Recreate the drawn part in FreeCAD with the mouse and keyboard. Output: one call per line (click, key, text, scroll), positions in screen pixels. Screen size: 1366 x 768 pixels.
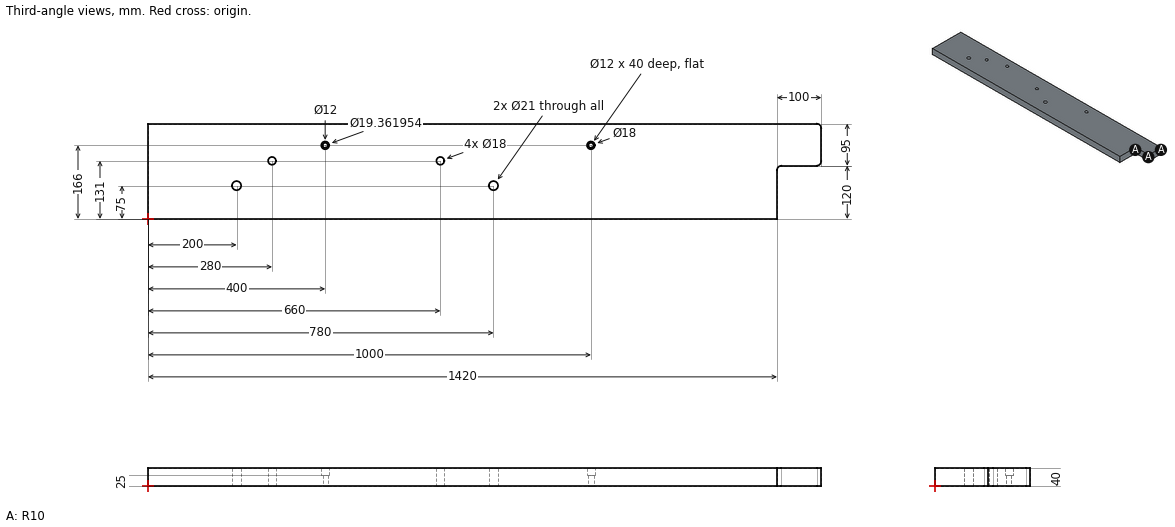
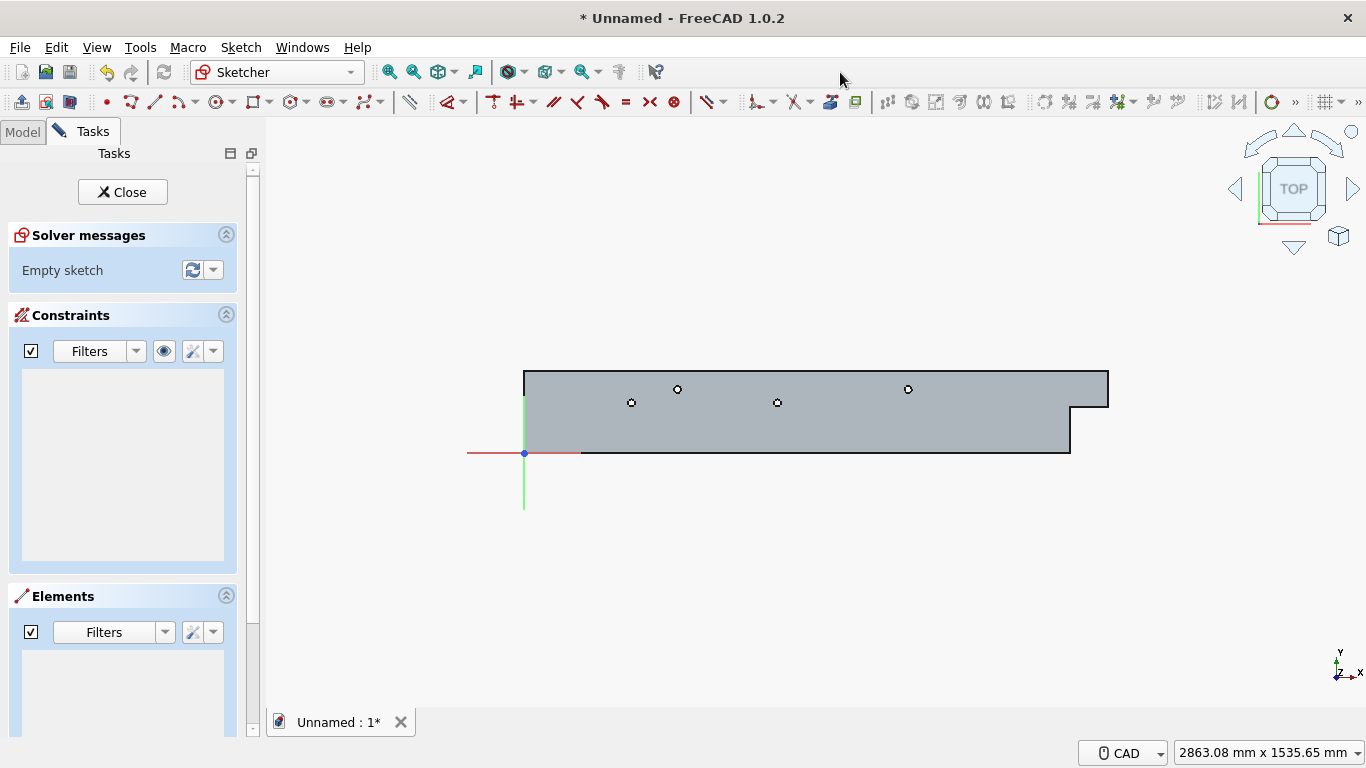
scroll(617, 457, up, 4)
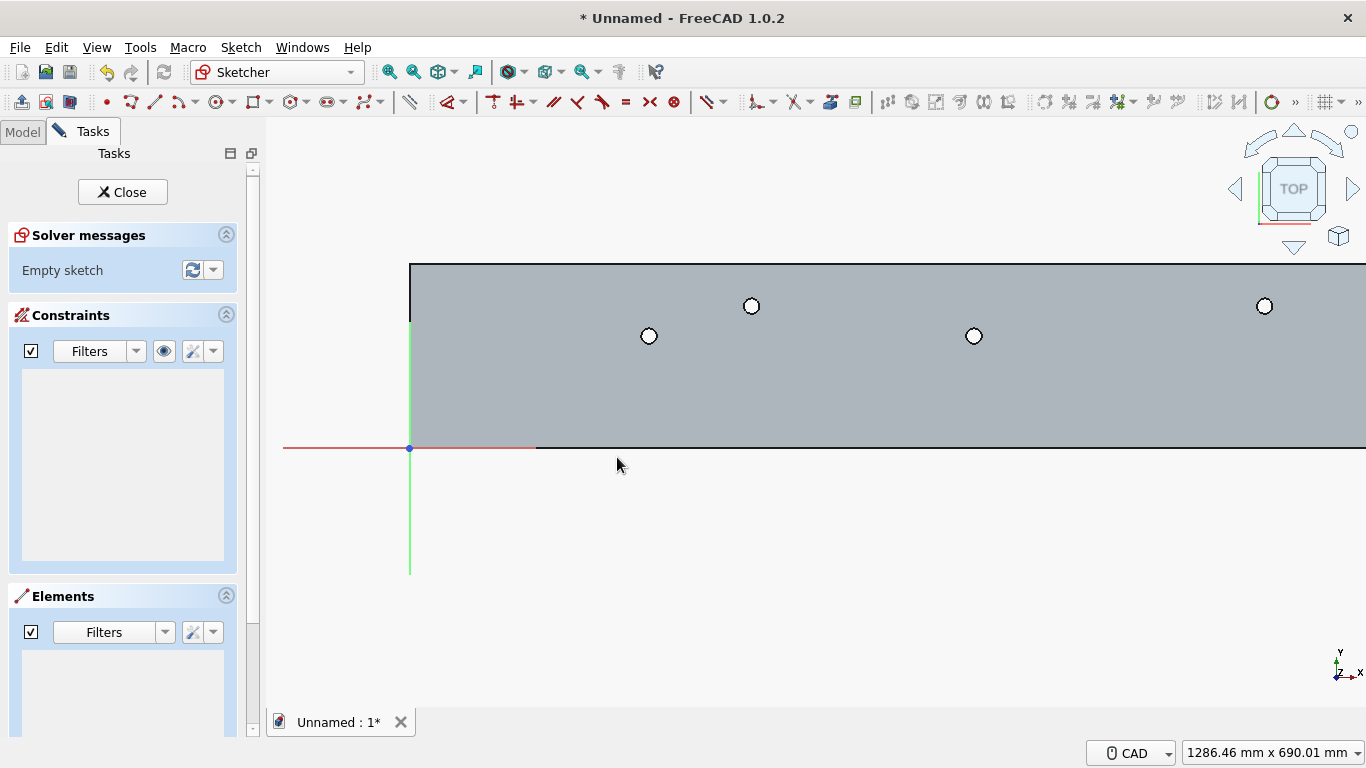
click(216, 102)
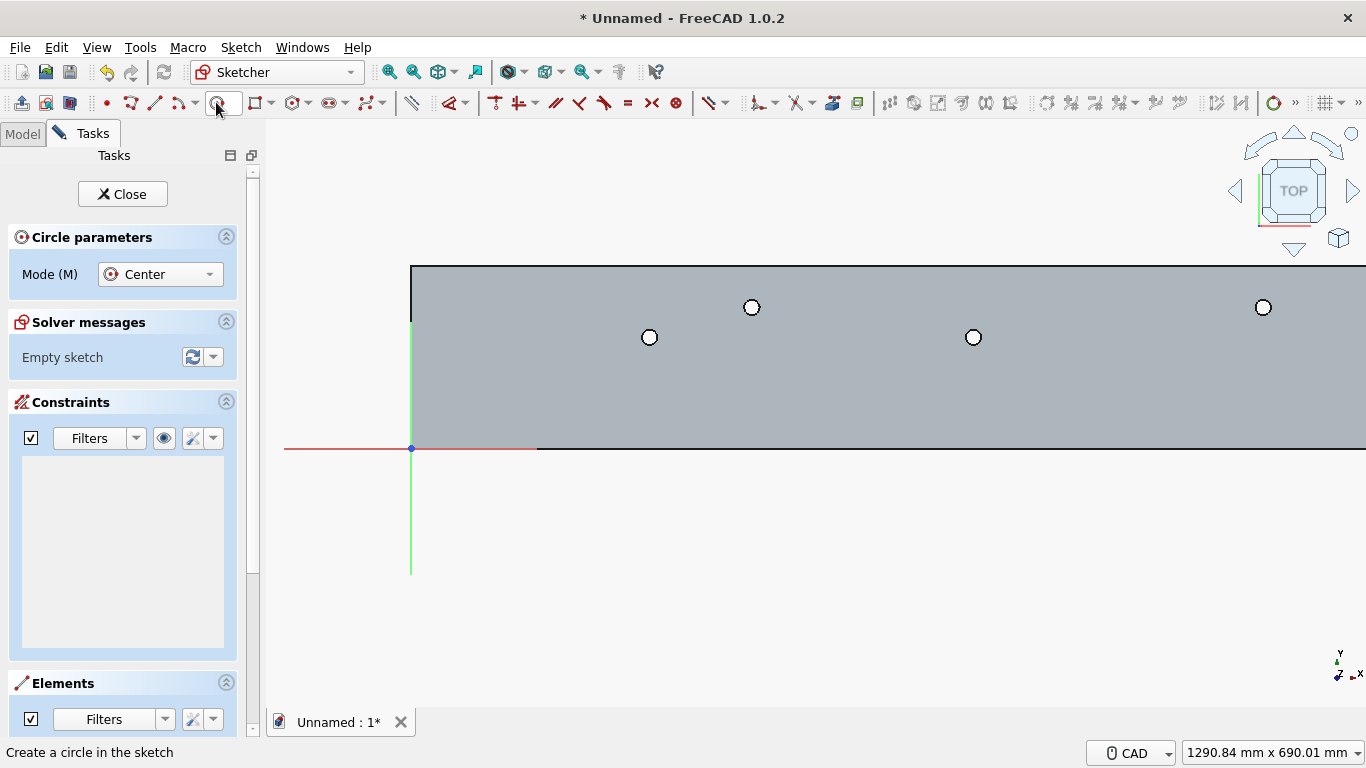
scroll(1076, 385, up, 5)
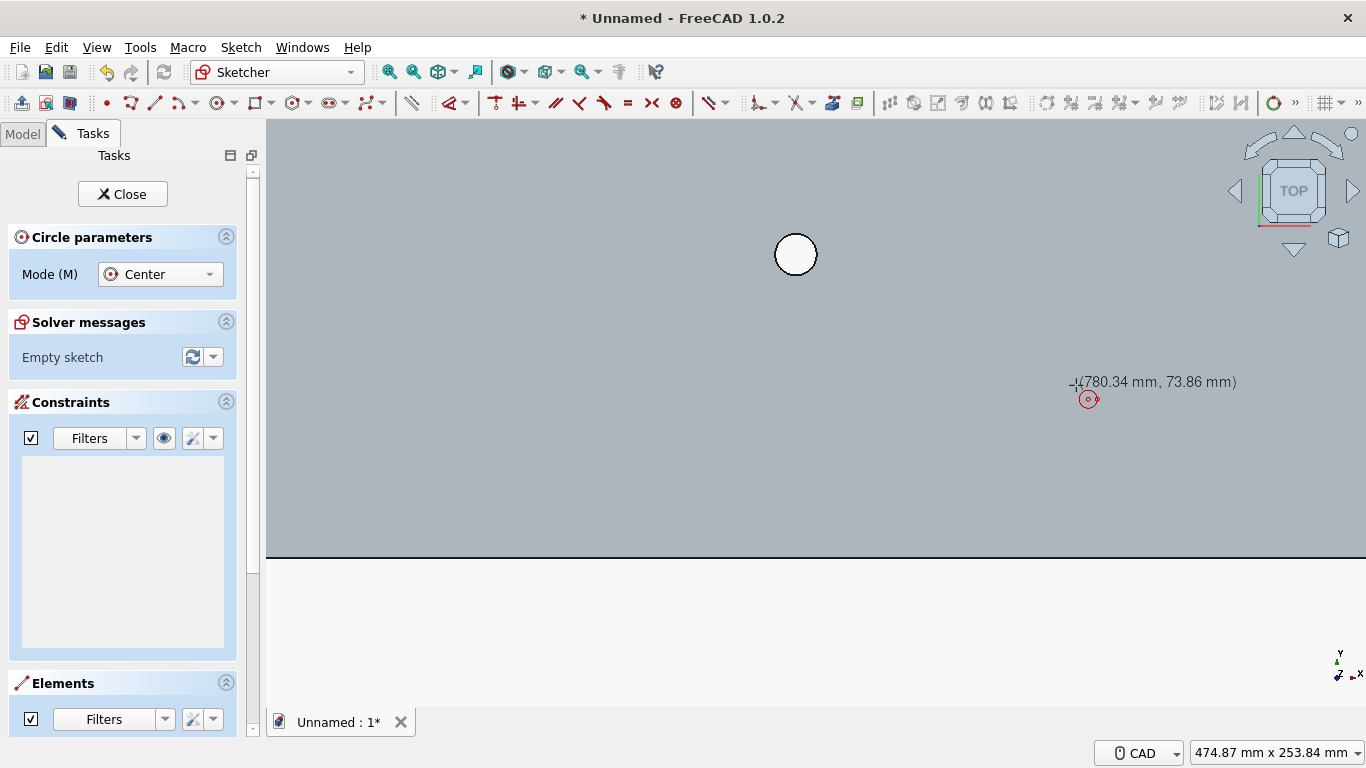
click(1074, 384)
click(1091, 367)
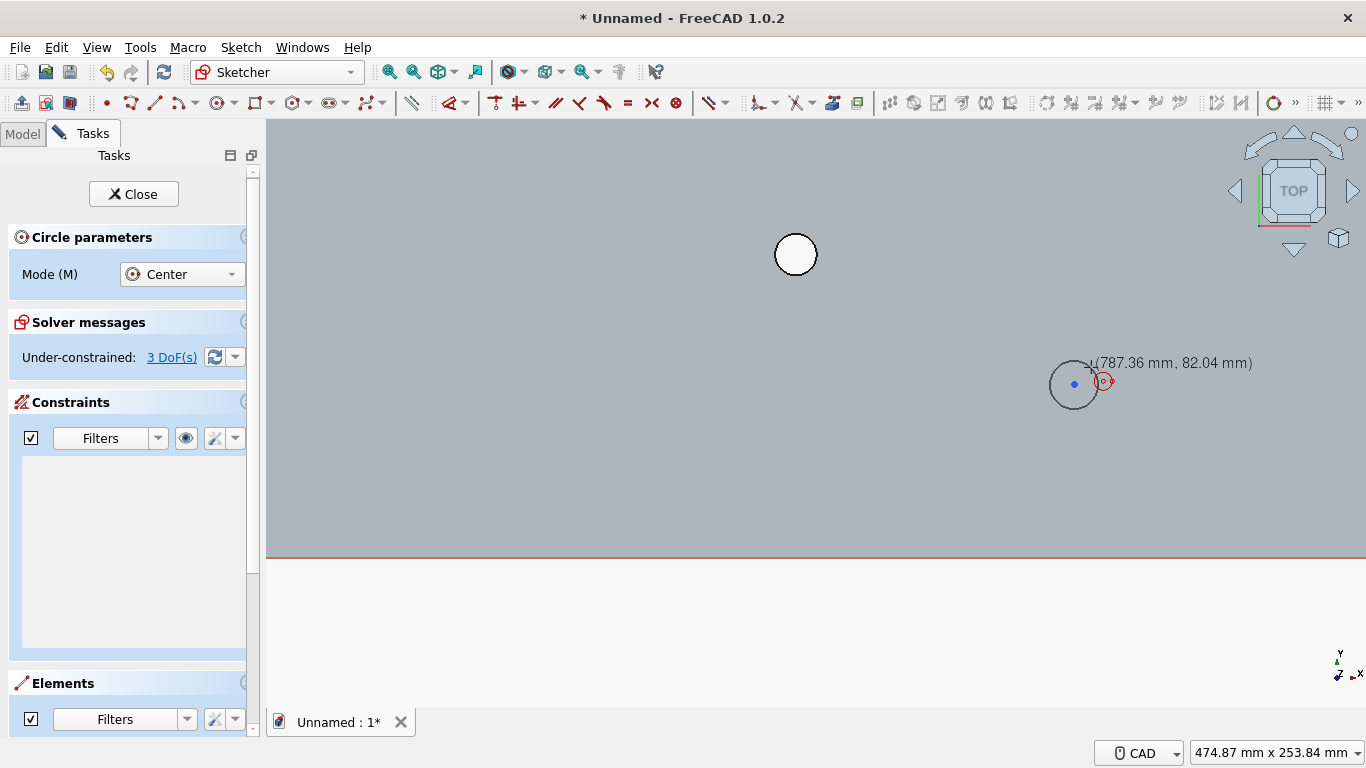
scroll(1076, 386, down, 5)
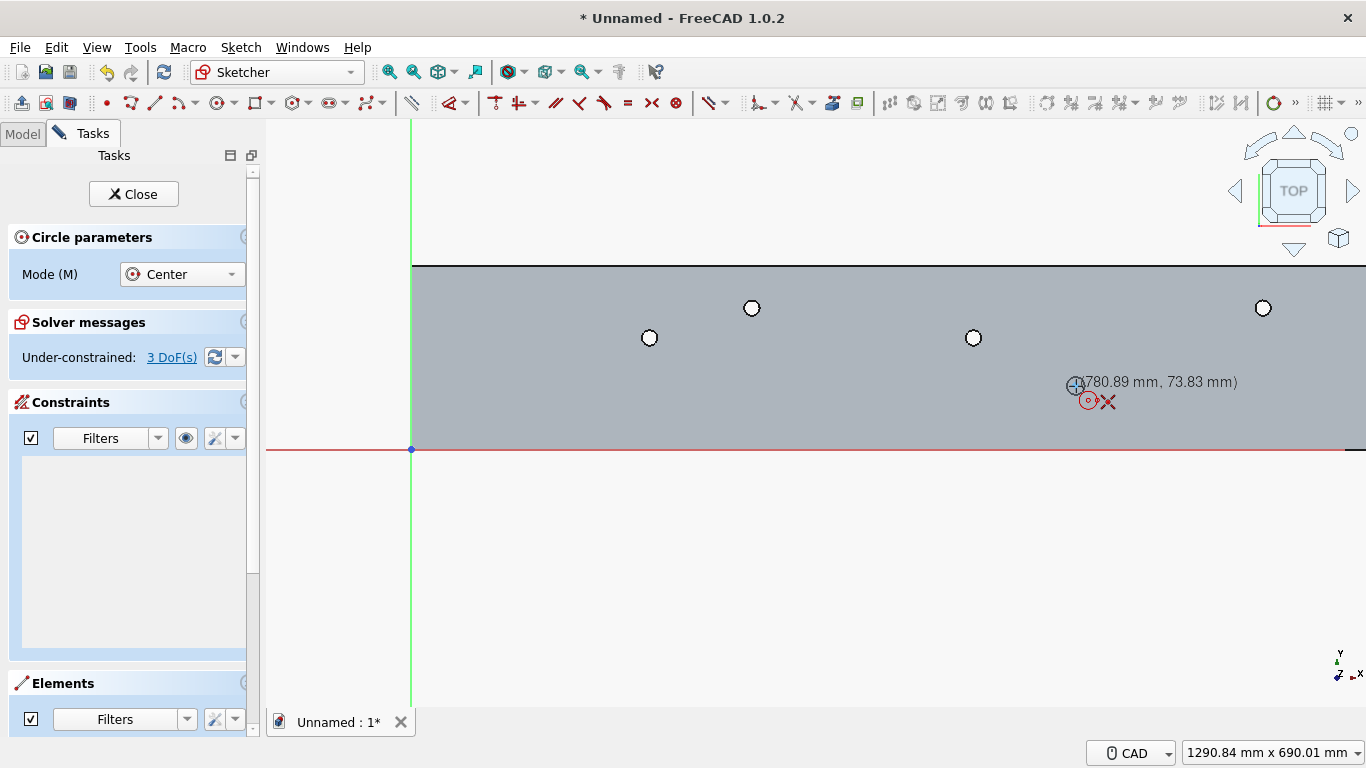
scroll(581, 386, up, 5)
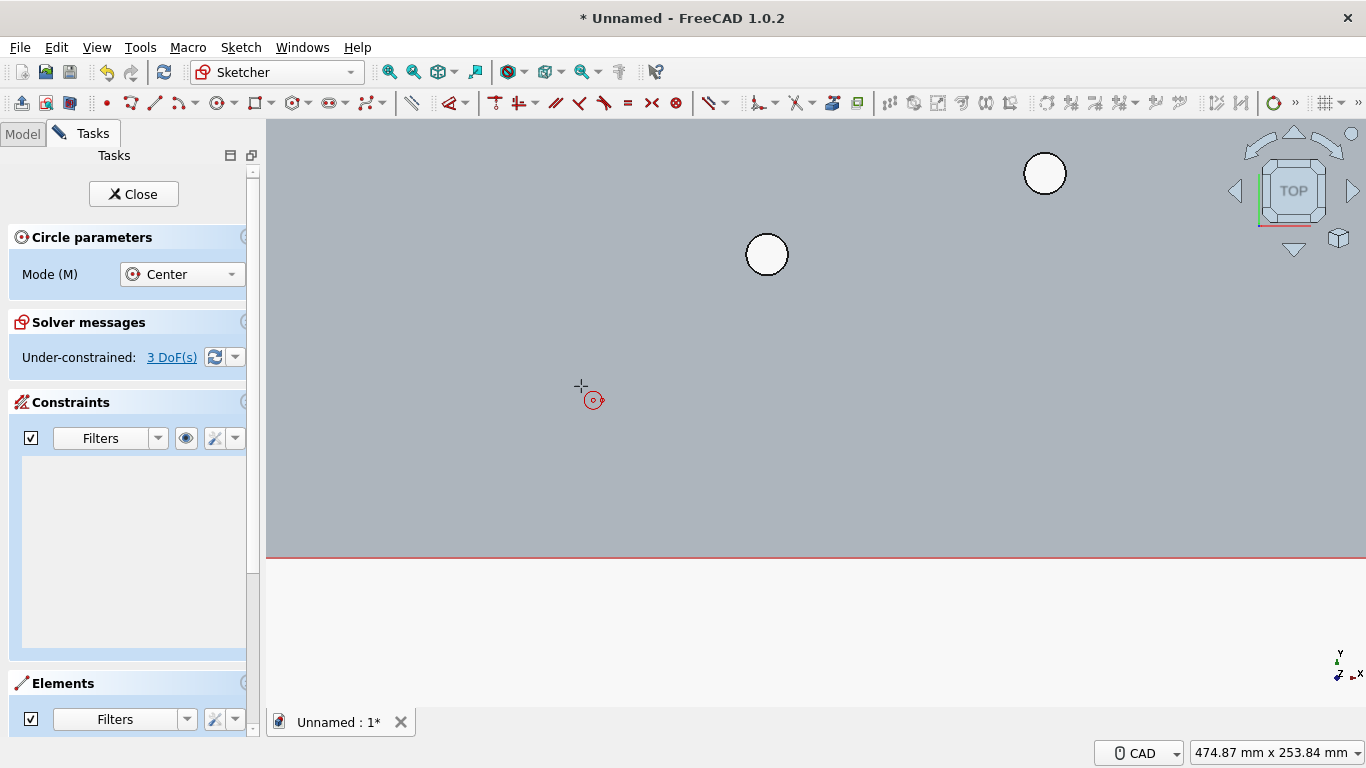
click(582, 384)
click(599, 367)
key(Escape)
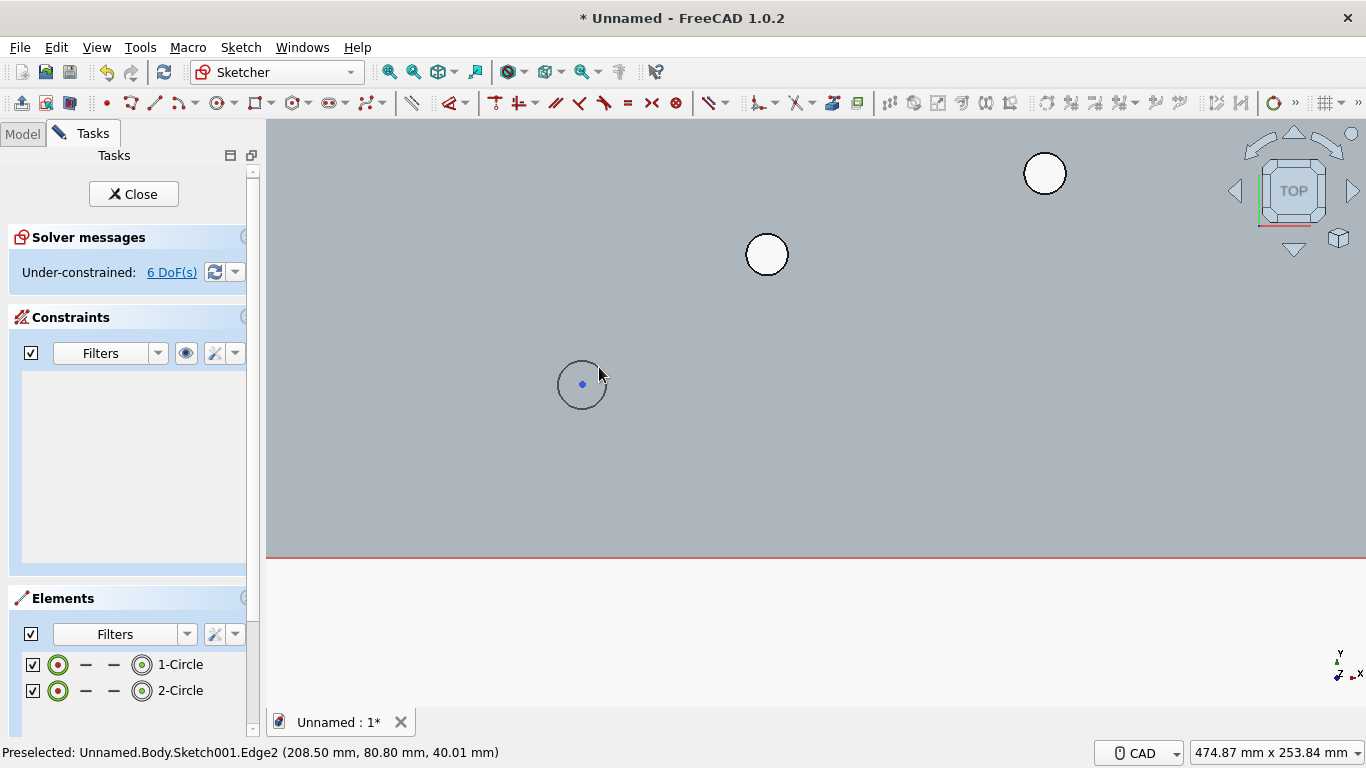
scroll(581, 386, down, 5)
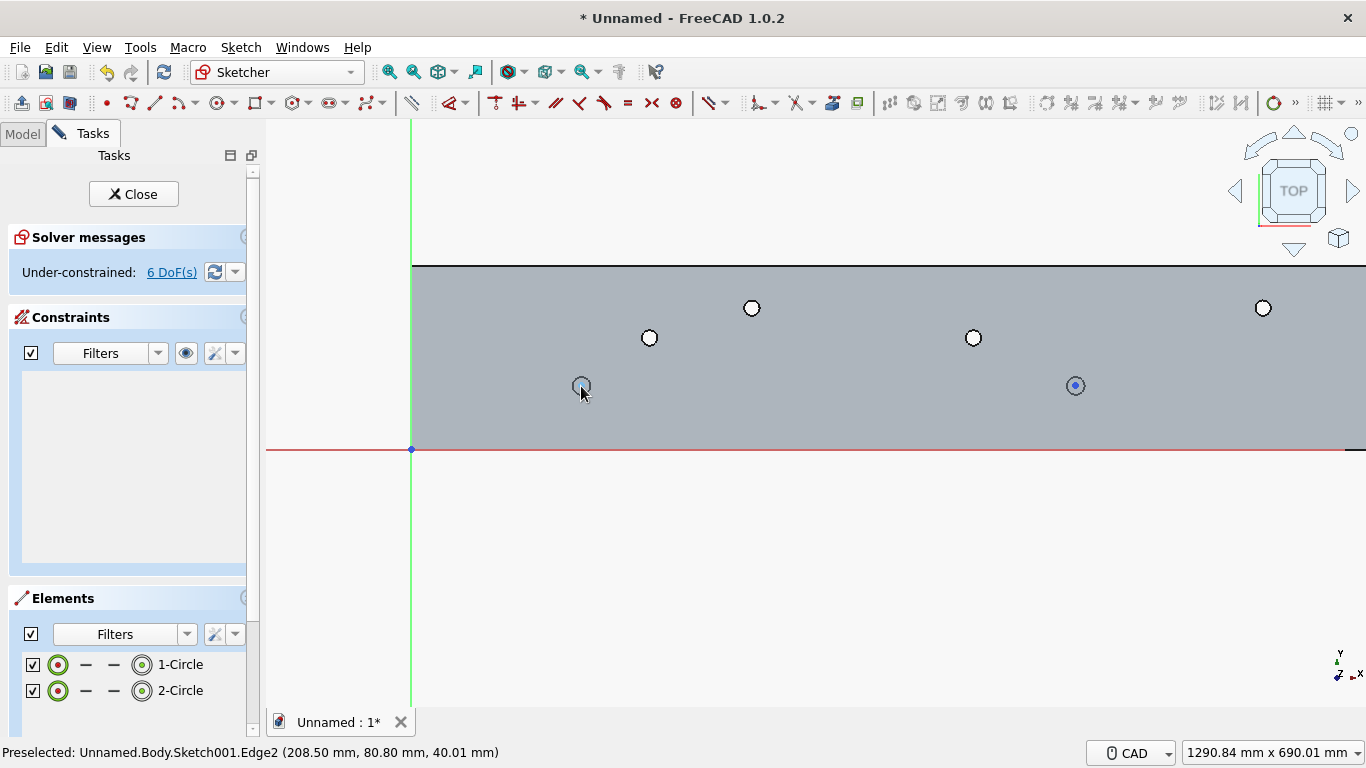
scroll(1082, 380, up, 3)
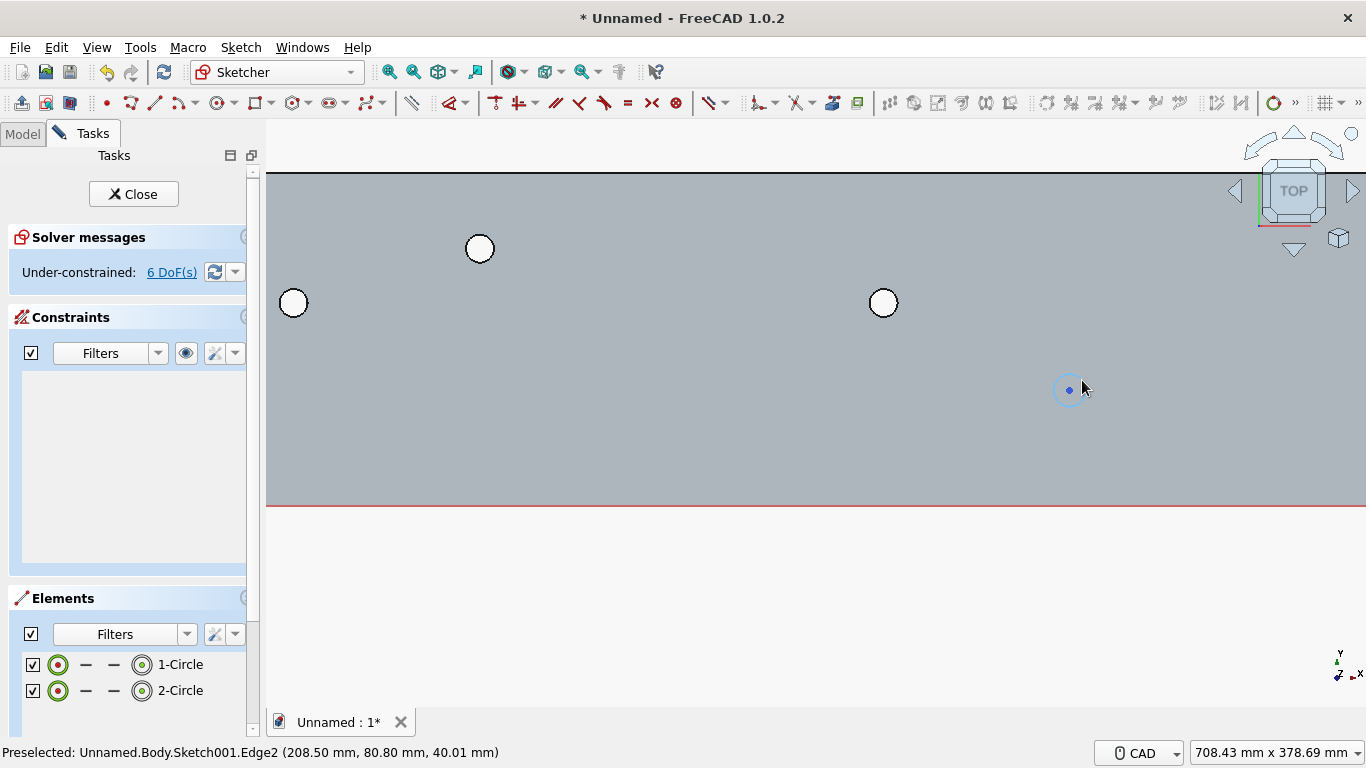
click(1081, 379)